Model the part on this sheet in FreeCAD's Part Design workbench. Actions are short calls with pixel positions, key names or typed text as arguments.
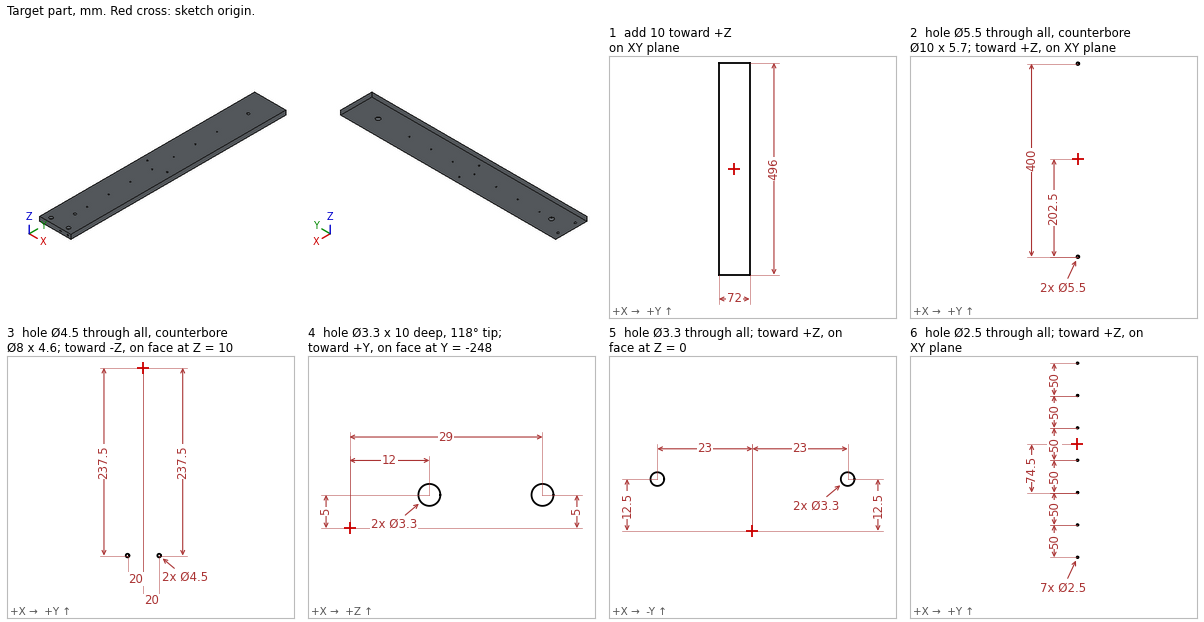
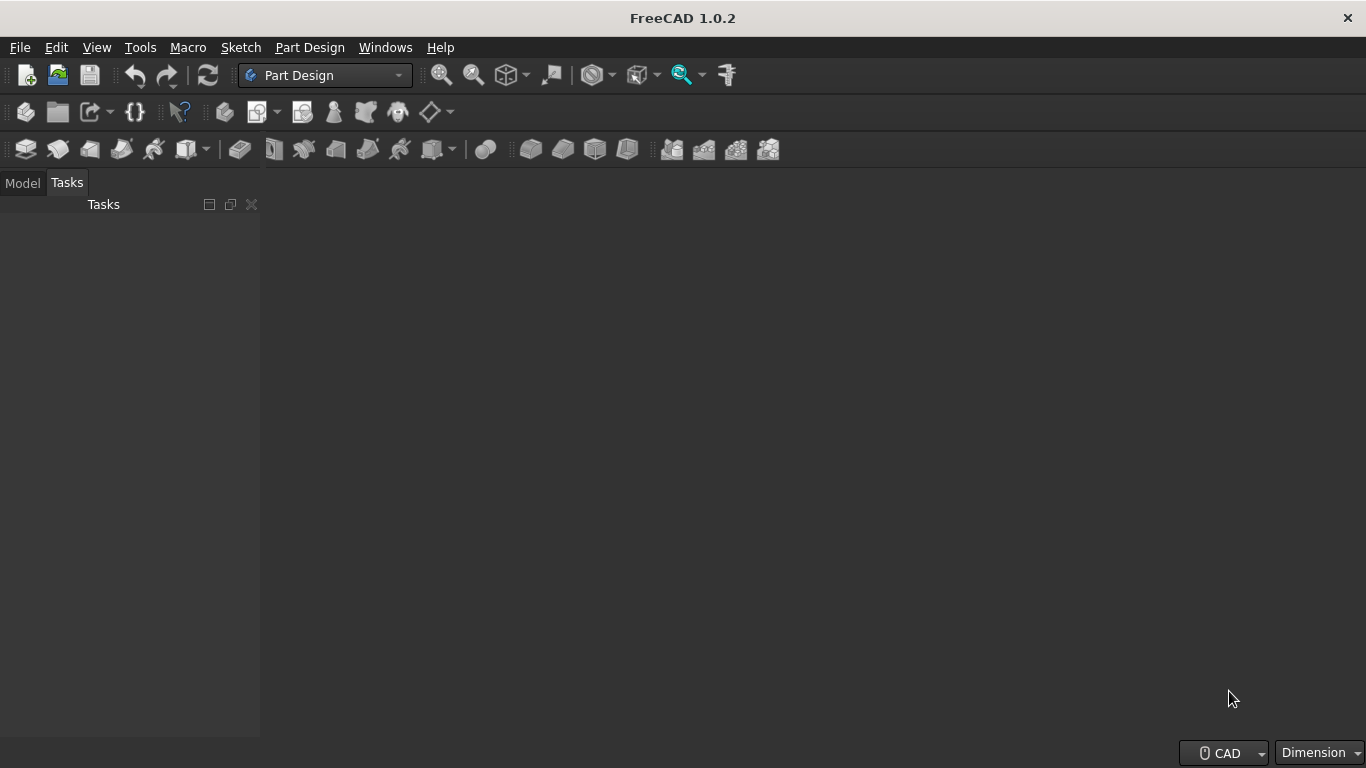
key(ctrl+n)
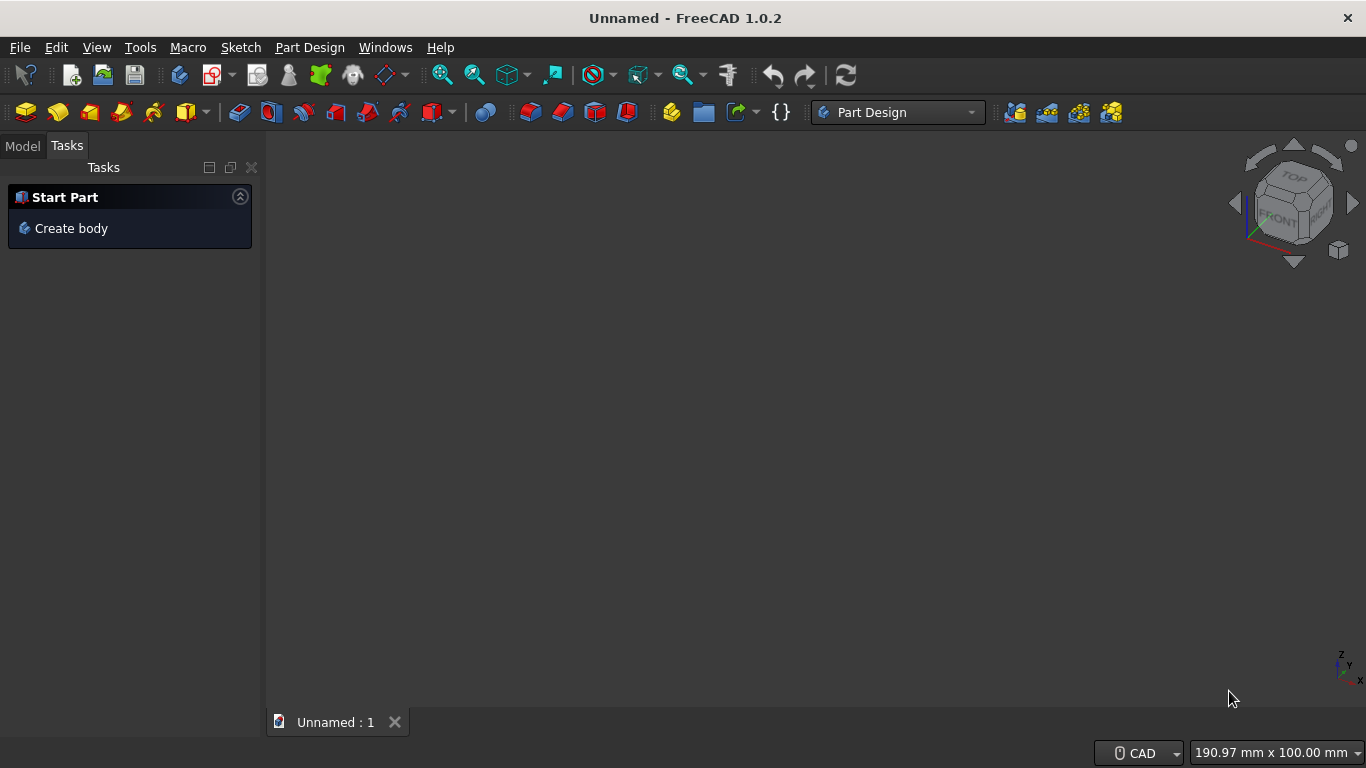
click(212, 76)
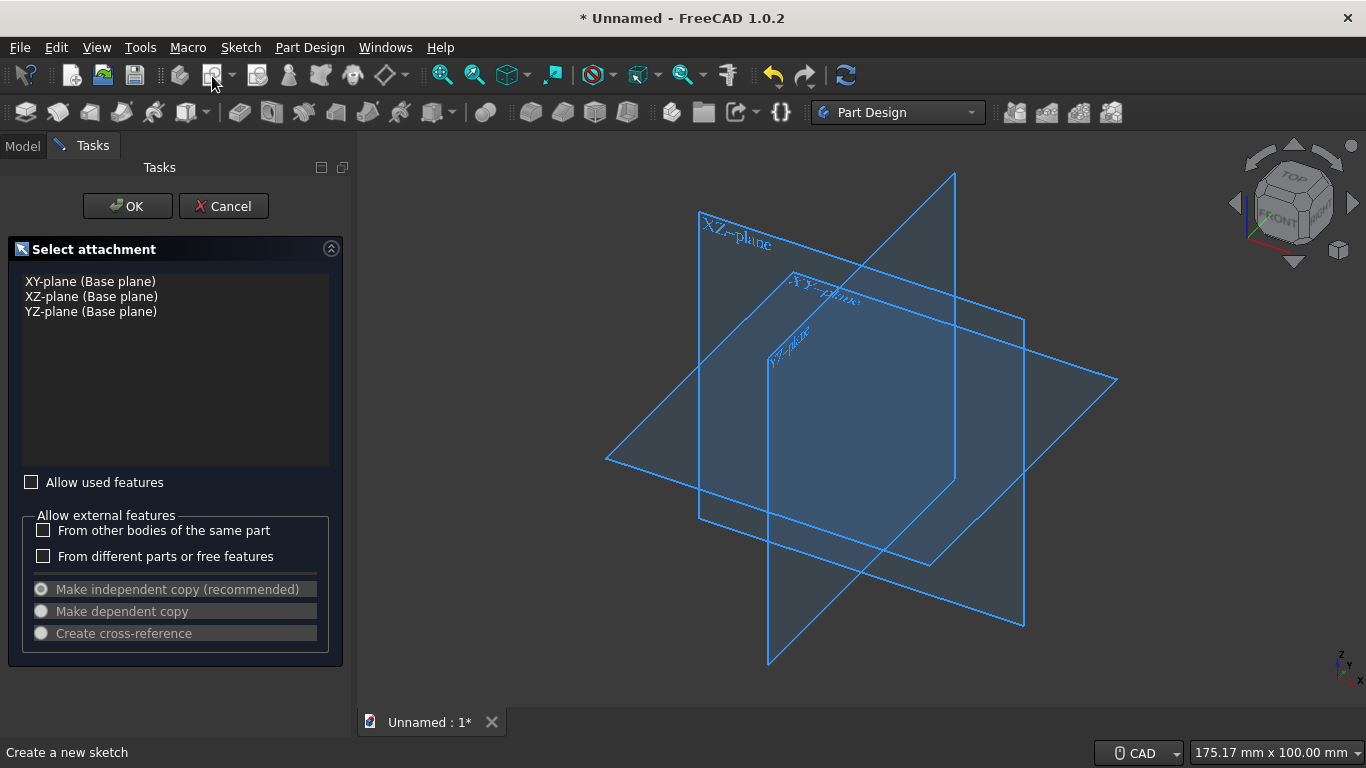
click(82, 282)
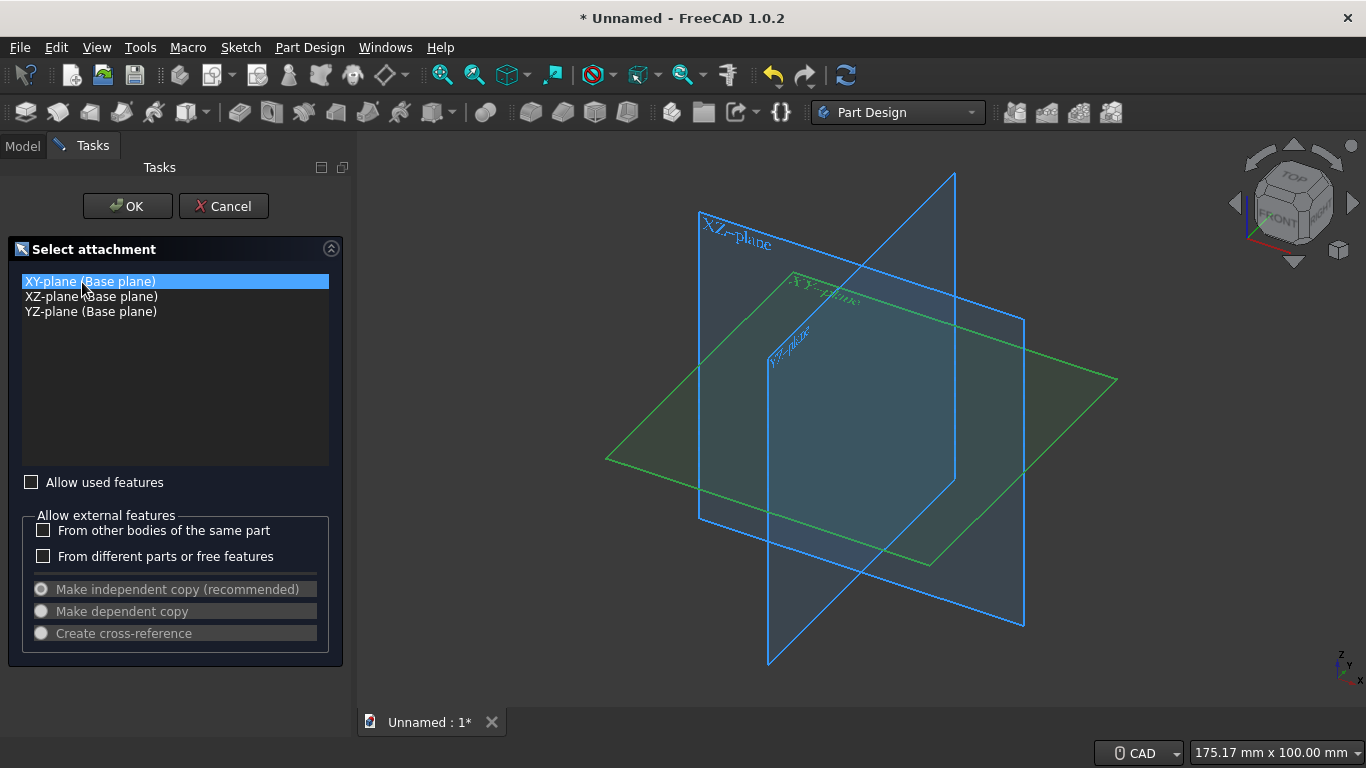
click(128, 206)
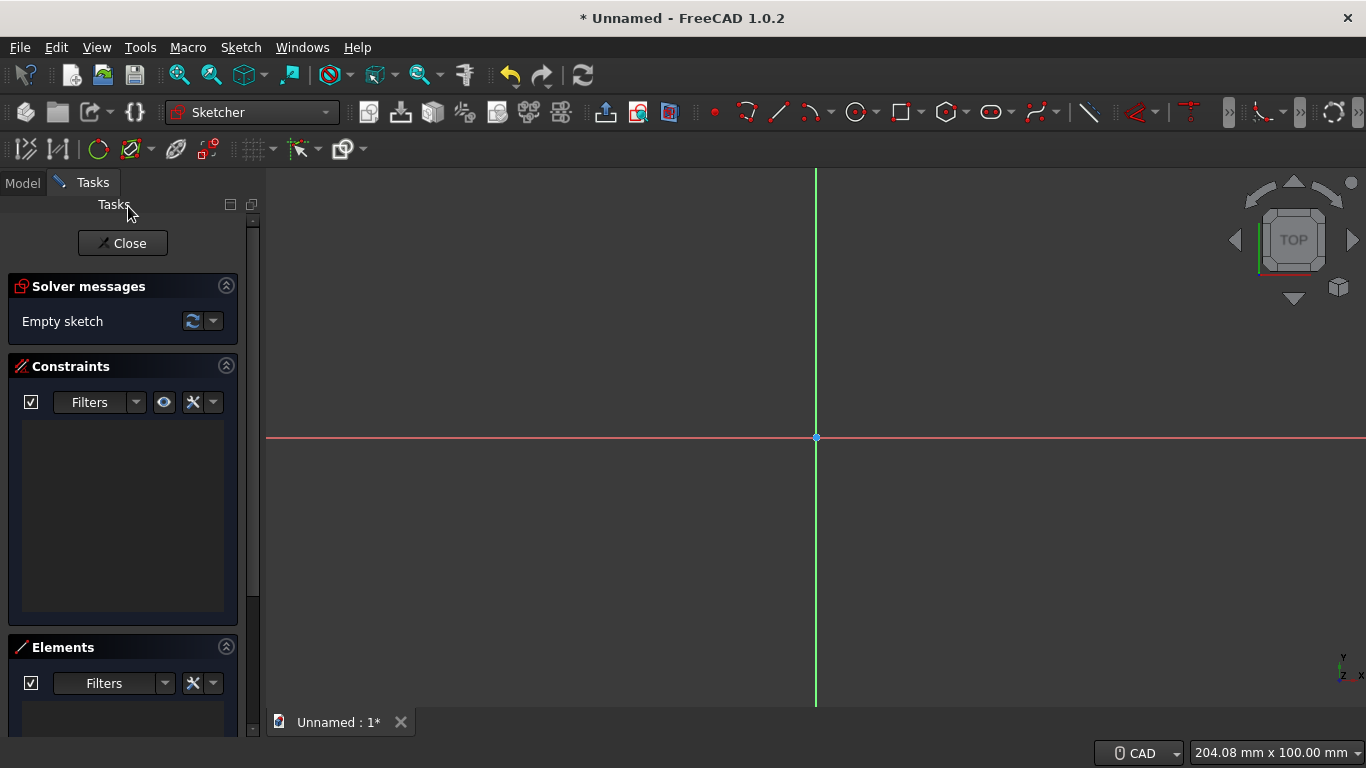
scroll(737, 438, down, 10)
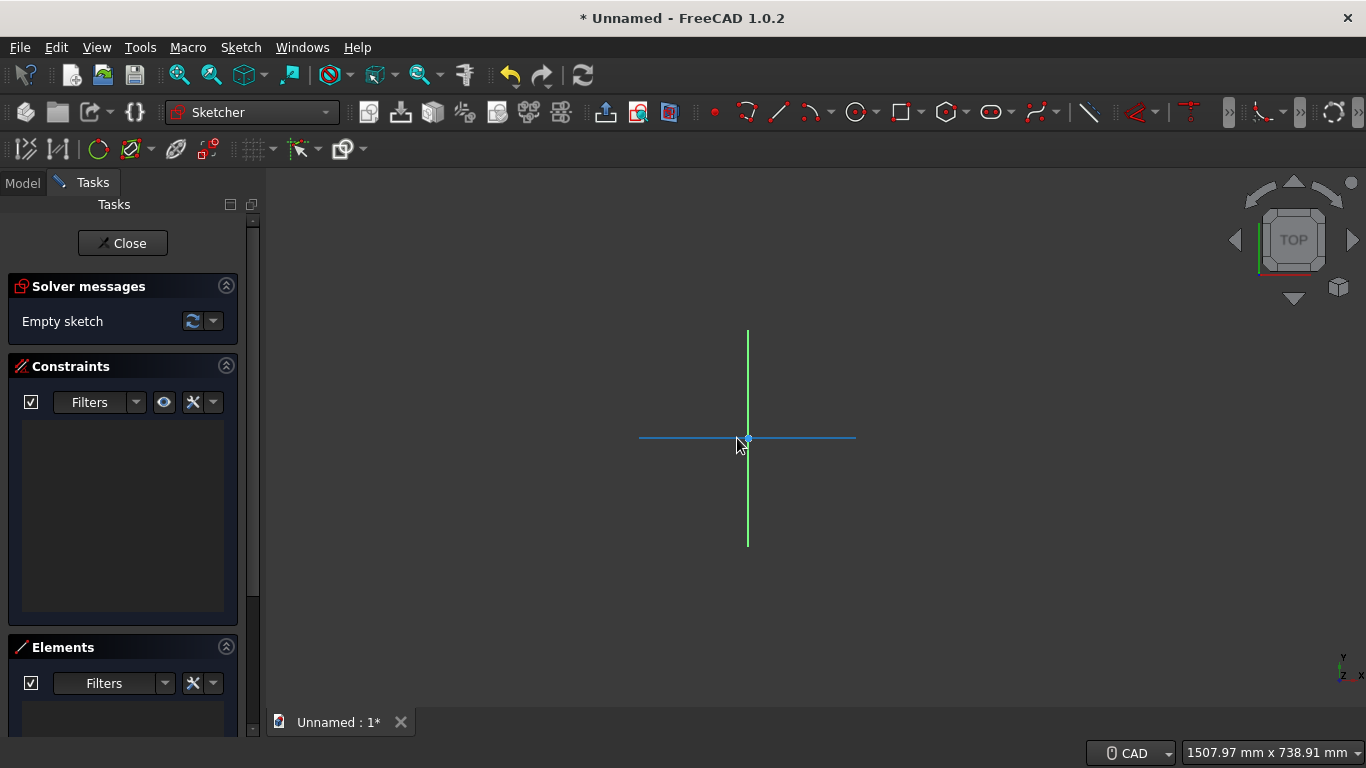
click(924, 112)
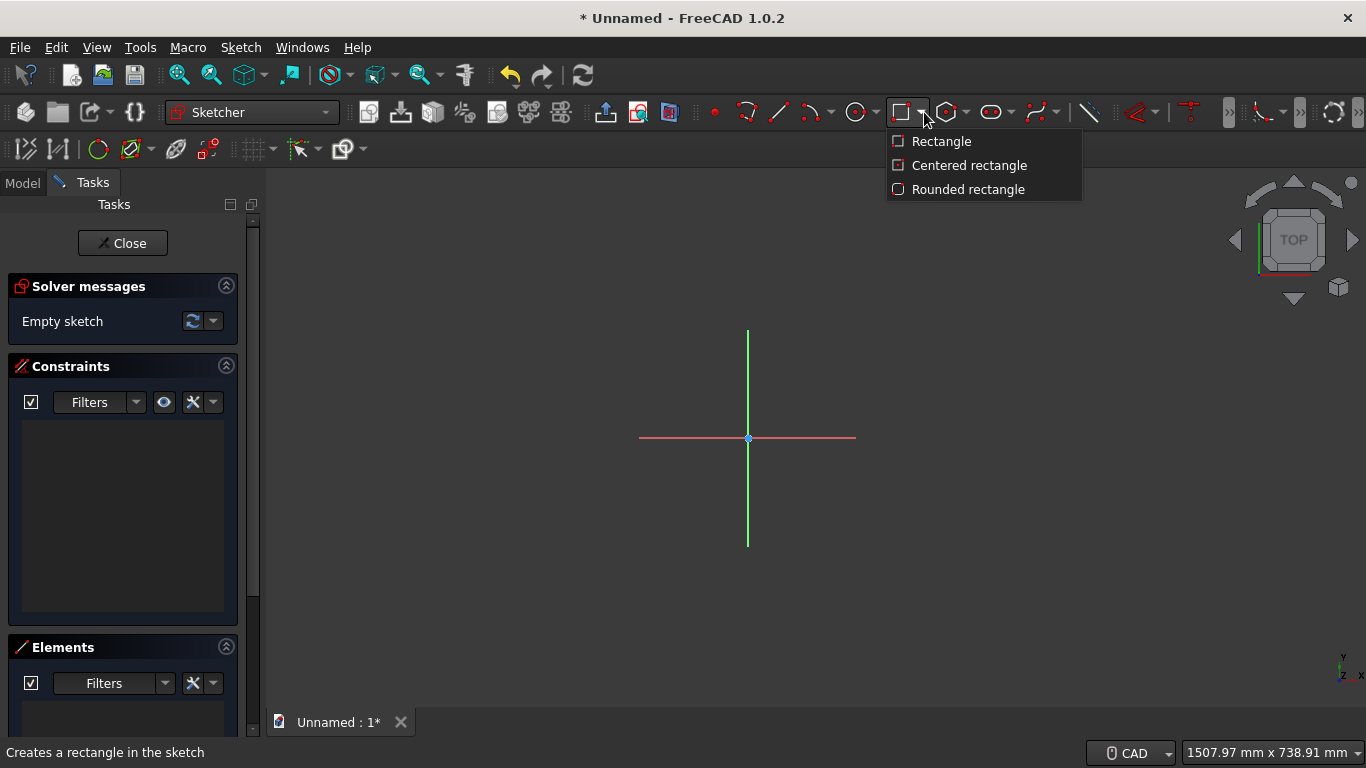
click(984, 165)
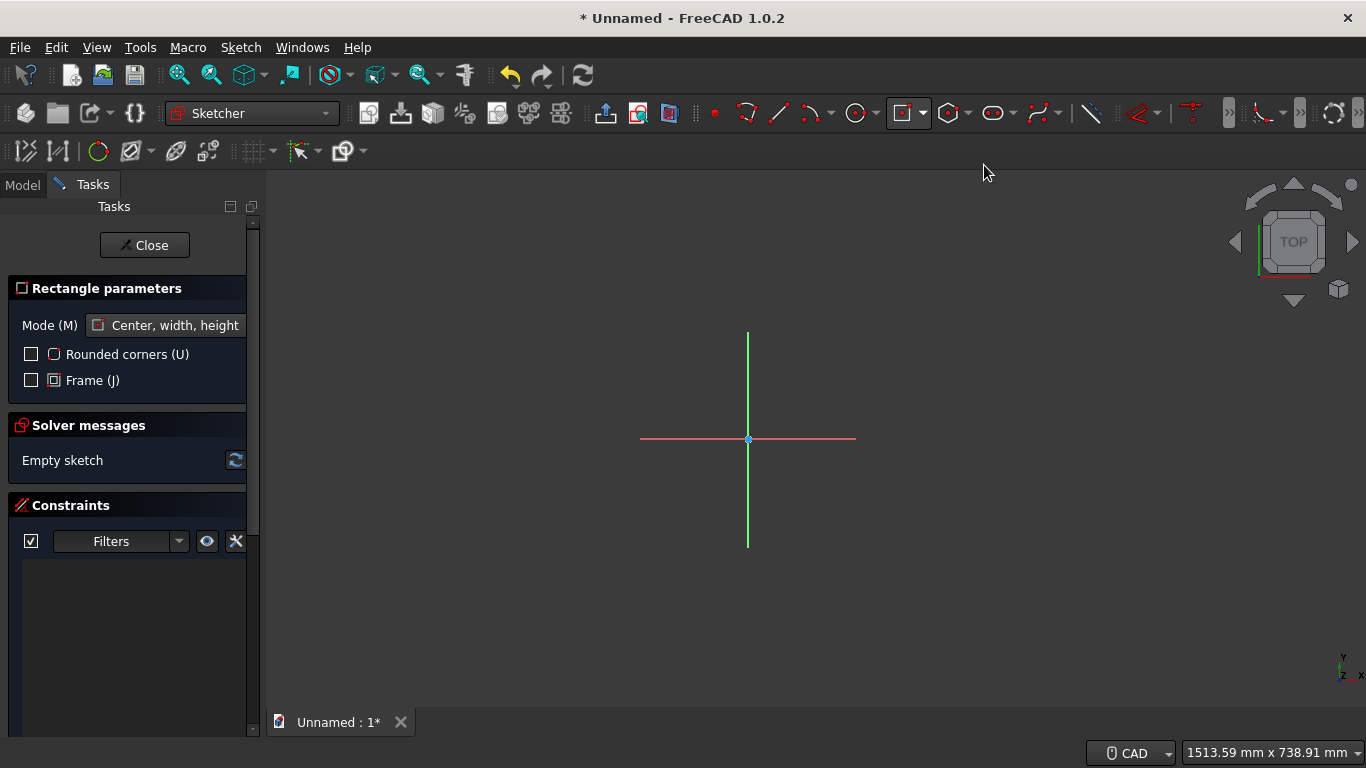
click(748, 439)
click(774, 259)
key(Escape)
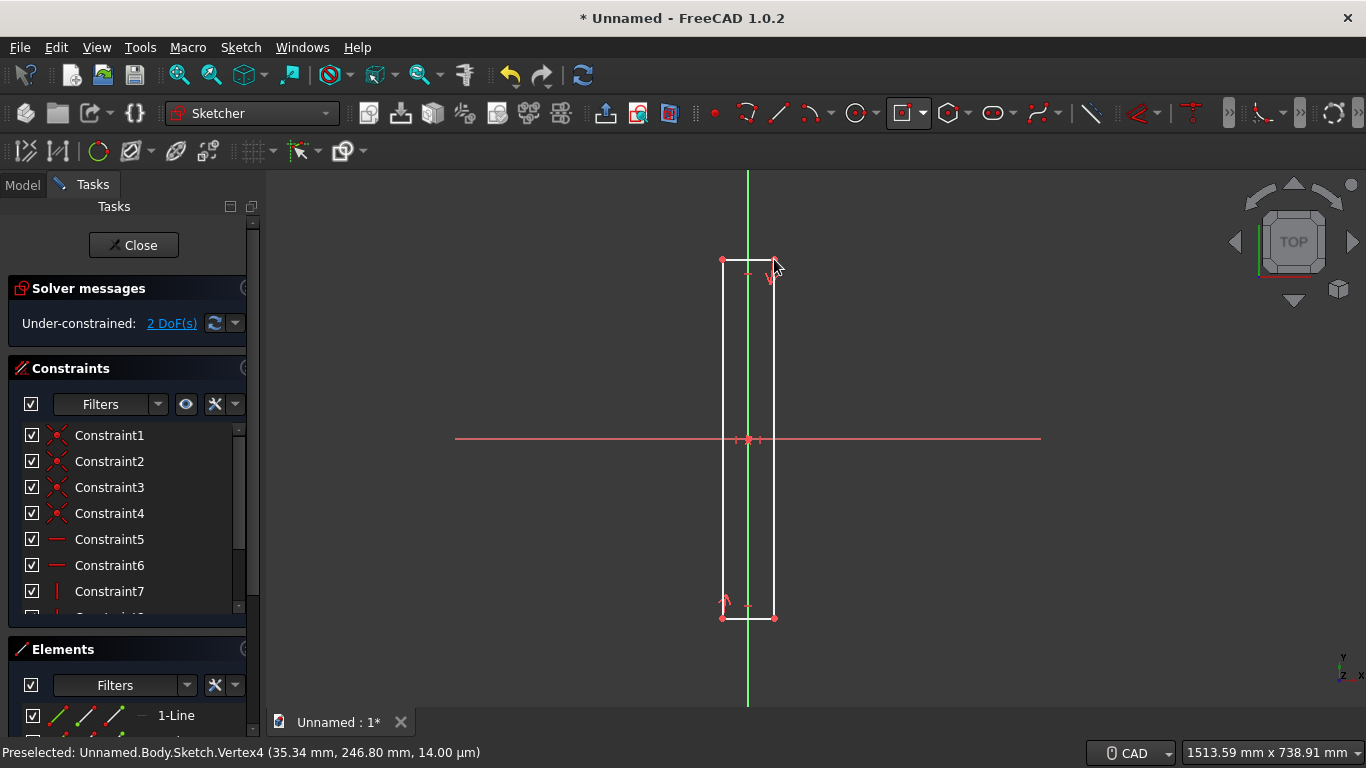
click(1138, 114)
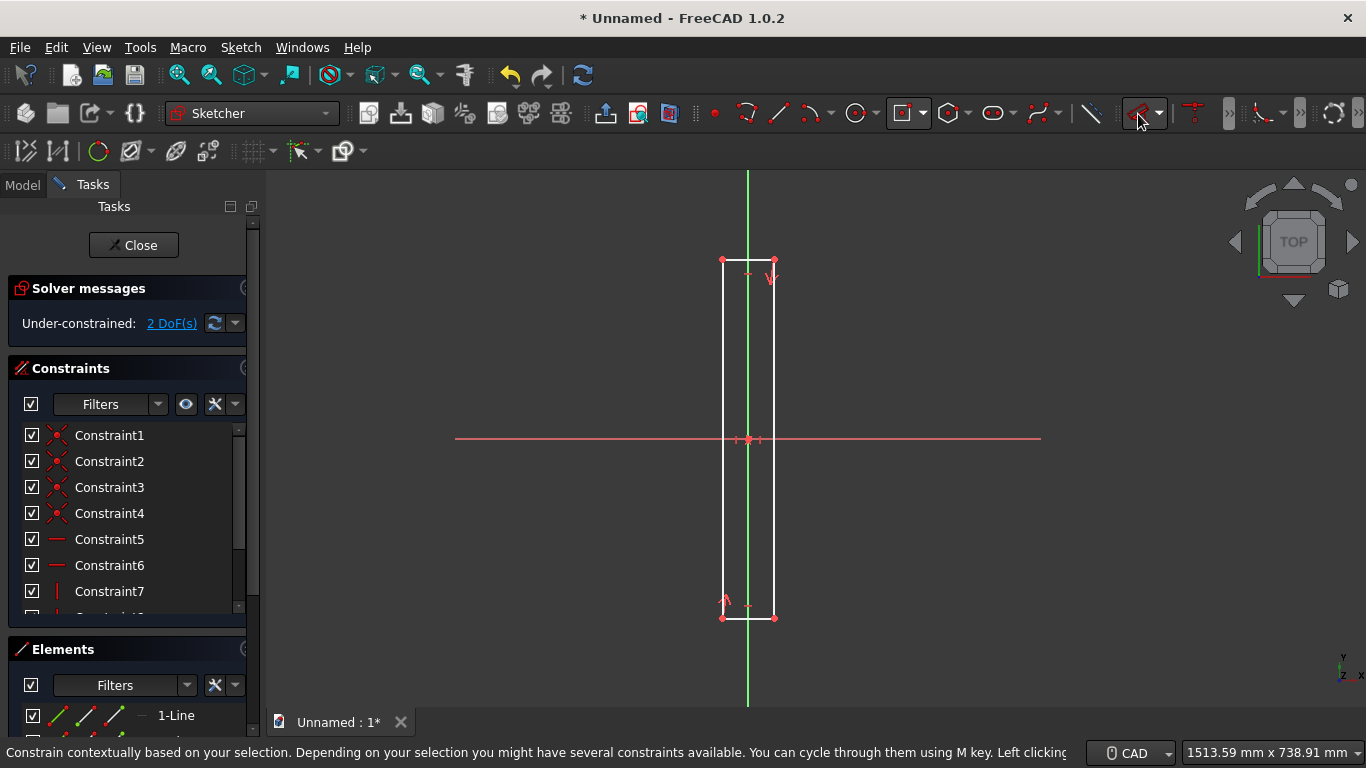
scroll(738, 619, up, 2)